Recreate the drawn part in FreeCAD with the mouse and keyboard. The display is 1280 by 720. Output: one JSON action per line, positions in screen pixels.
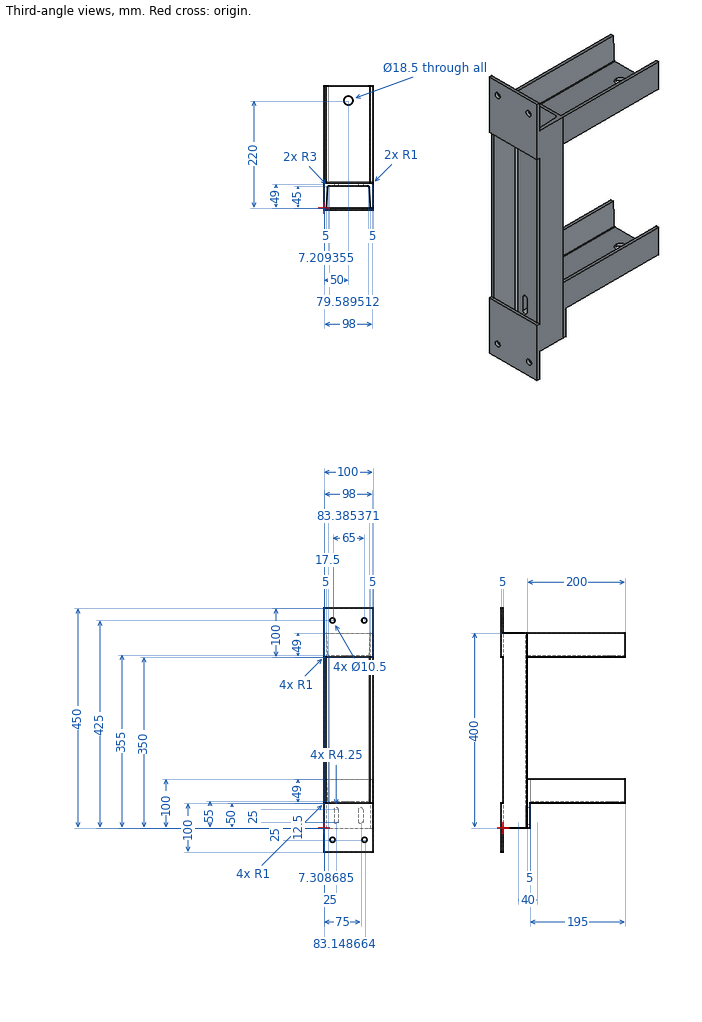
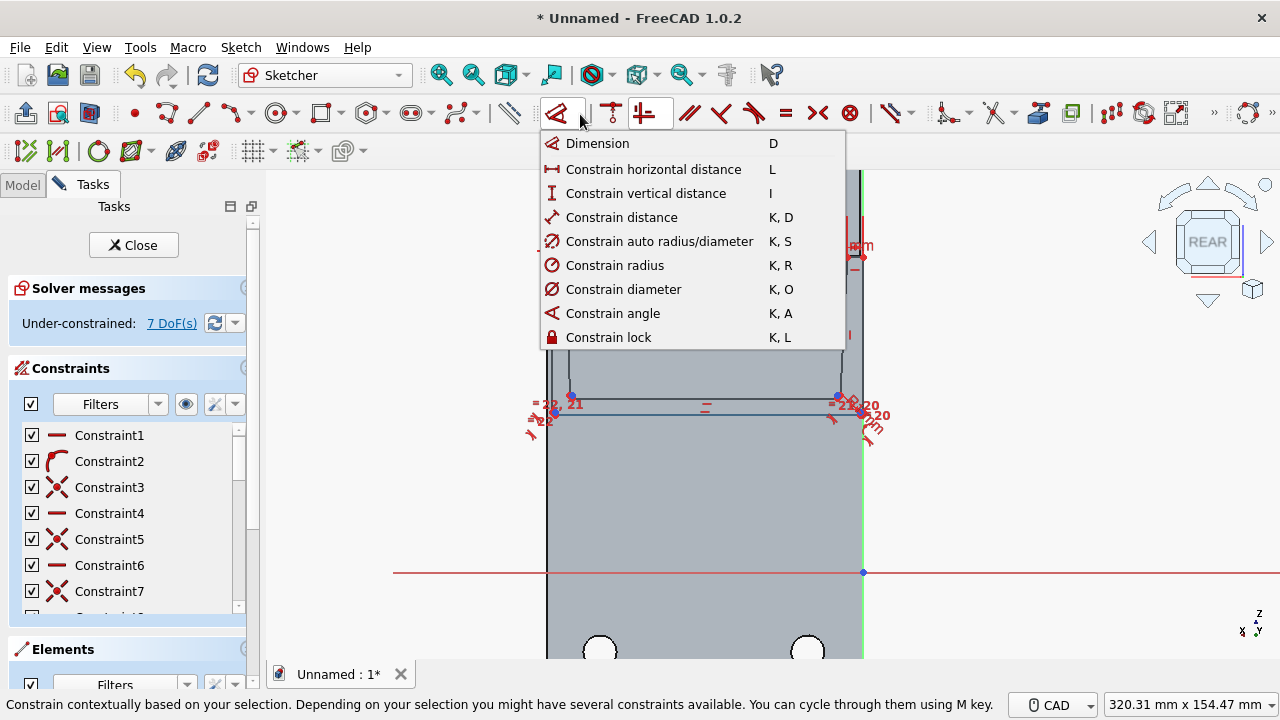
{"action": "left_click", "coordinate": [693, 169]}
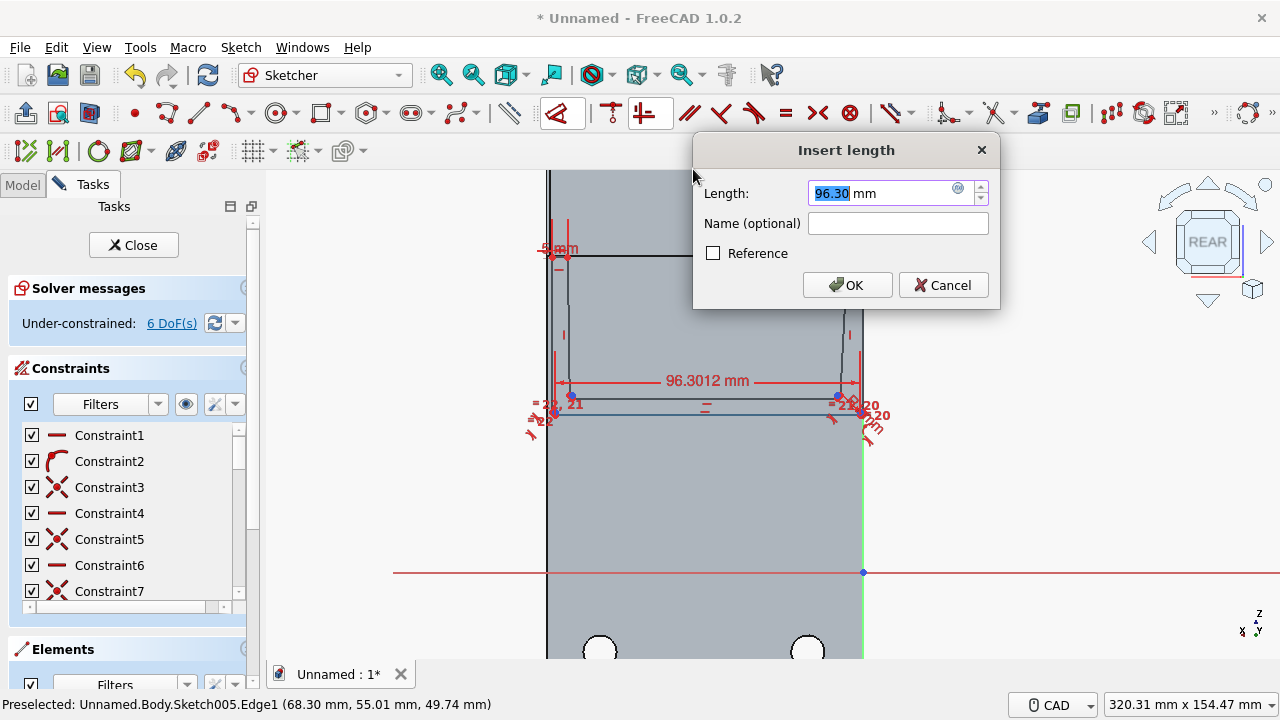
{"action": "type", "text": "98"}
{"action": "key", "text": "Return"}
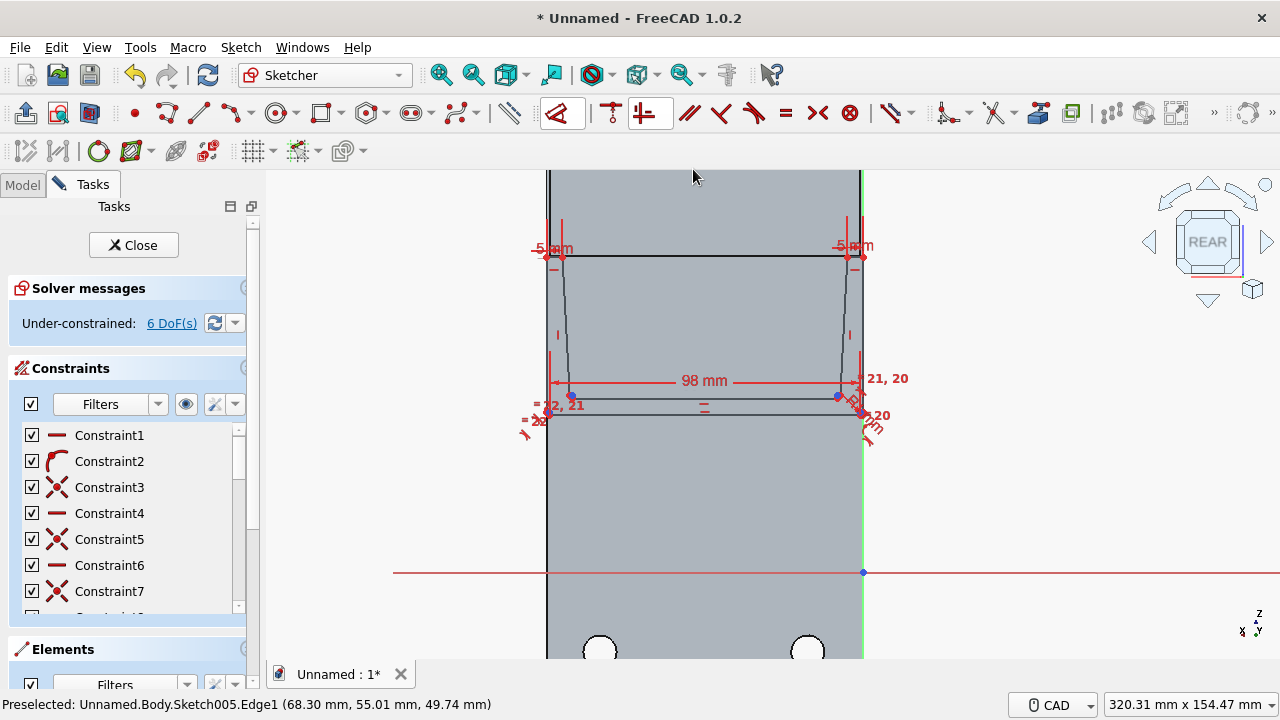
{"action": "left_click", "coordinate": [863, 366]}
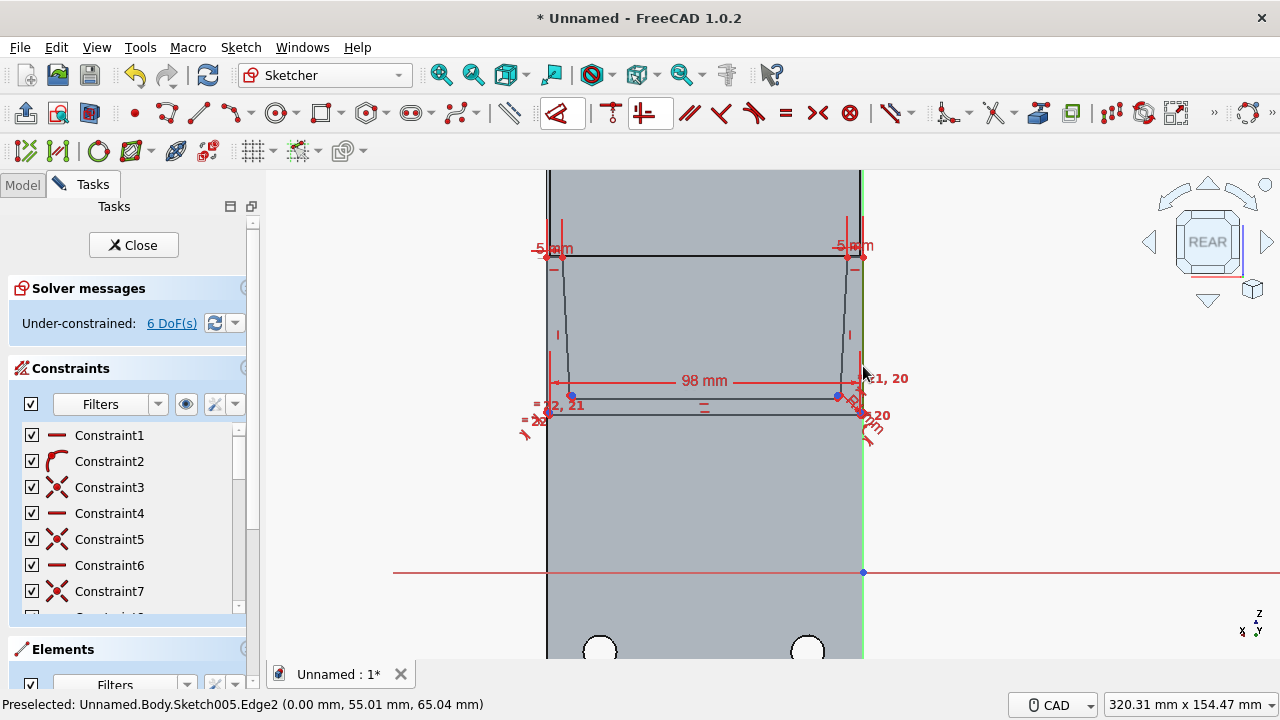
{"action": "key", "text": "i"}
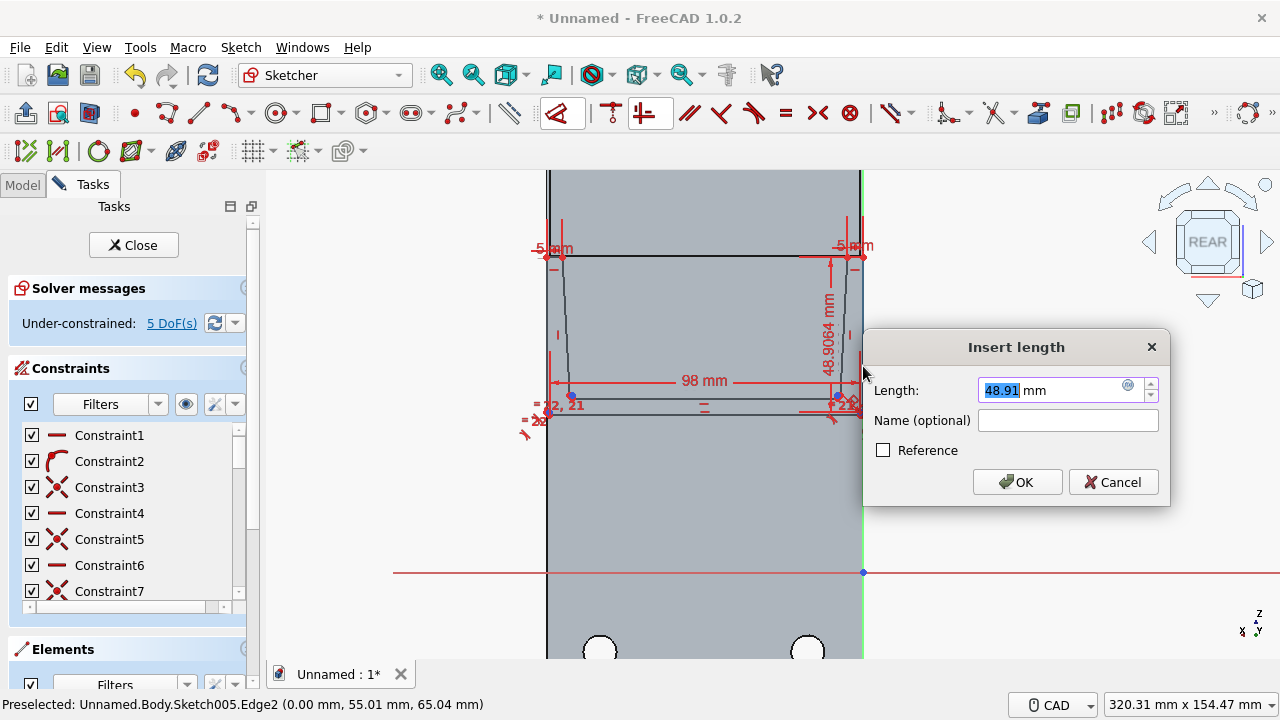
{"action": "type", "text": "49"}
{"action": "key", "text": "Return"}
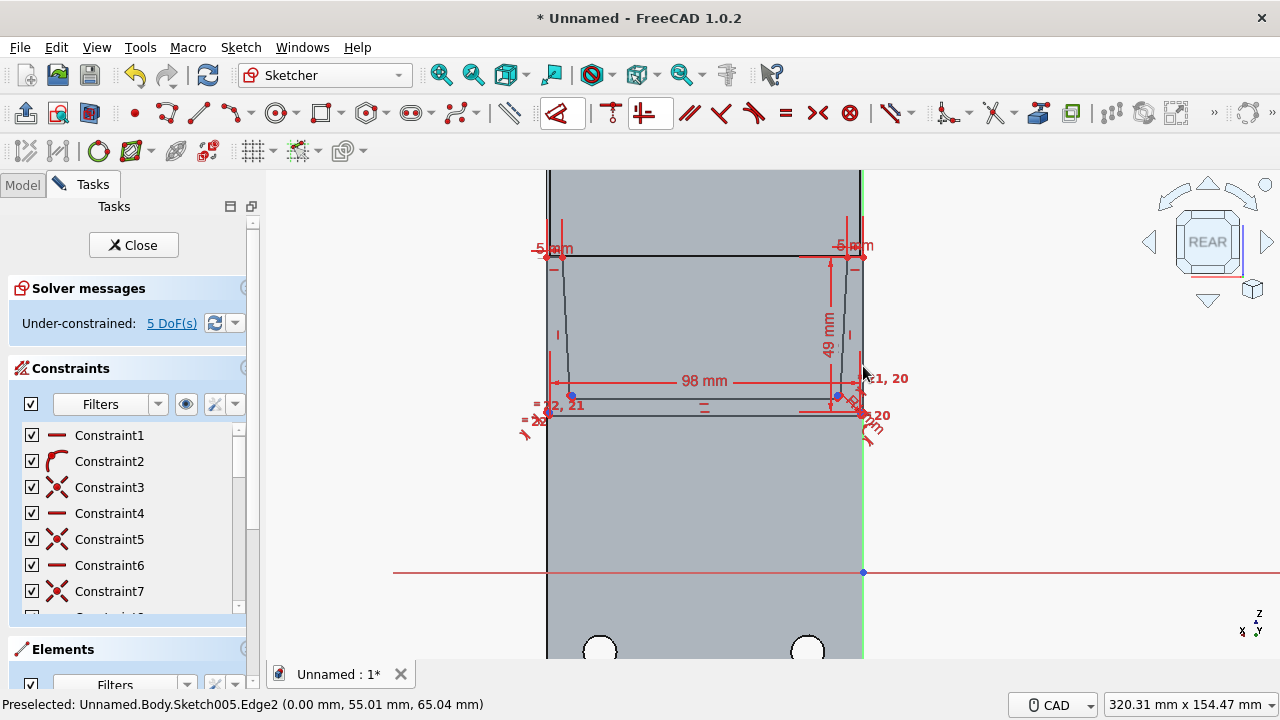
{"action": "left_click", "coordinate": [547, 304]}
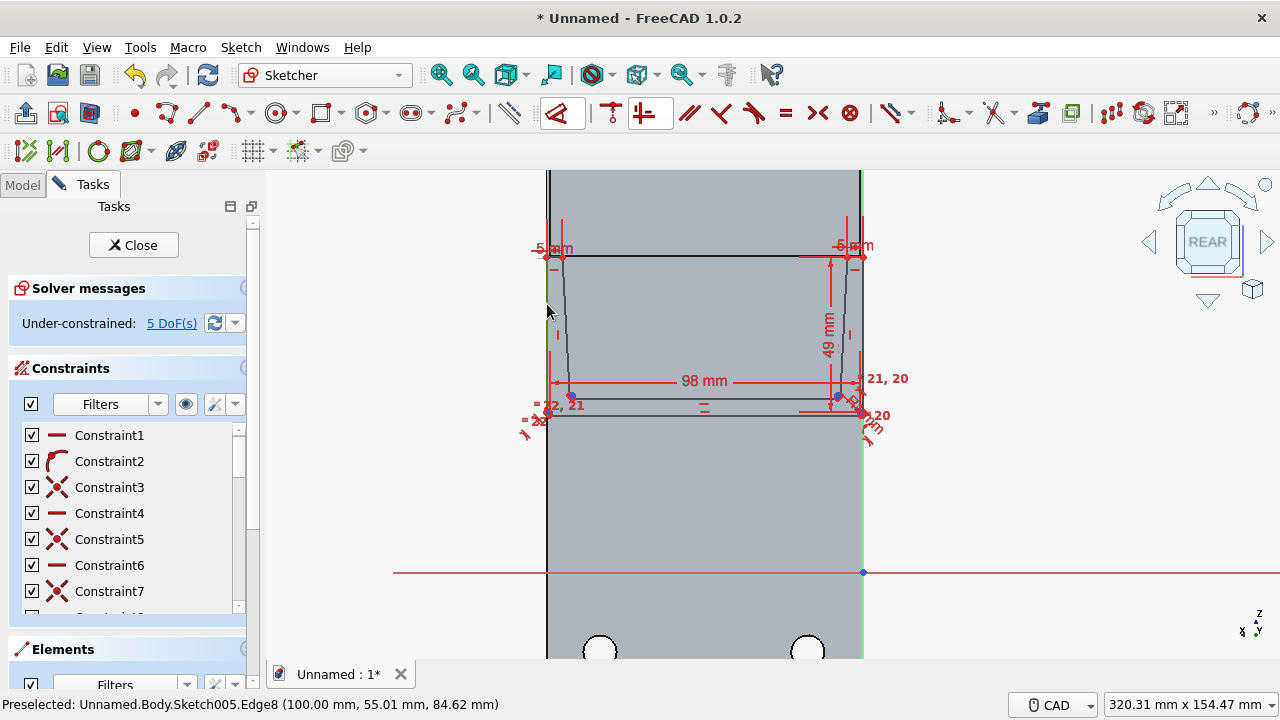
{"action": "left_click", "coordinate": [580, 114]}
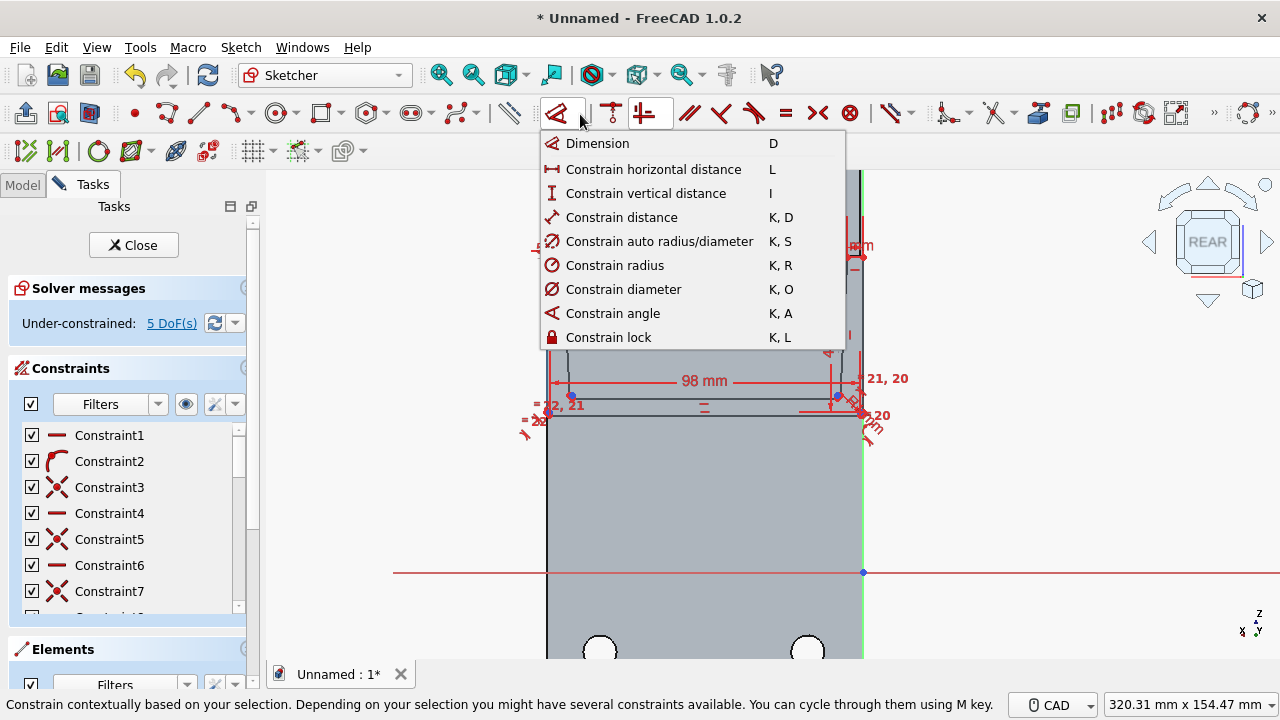
{"action": "left_click", "coordinate": [693, 193]}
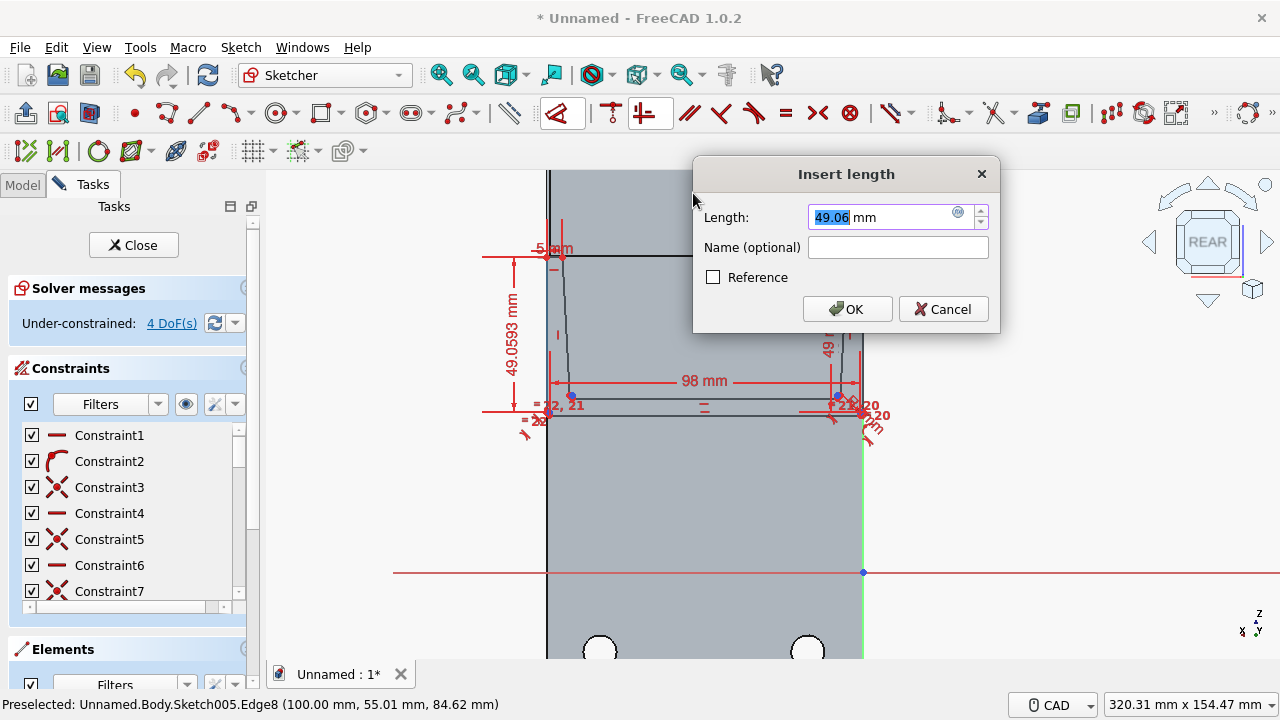
{"action": "type", "text": "49"}
{"action": "key", "text": "Return"}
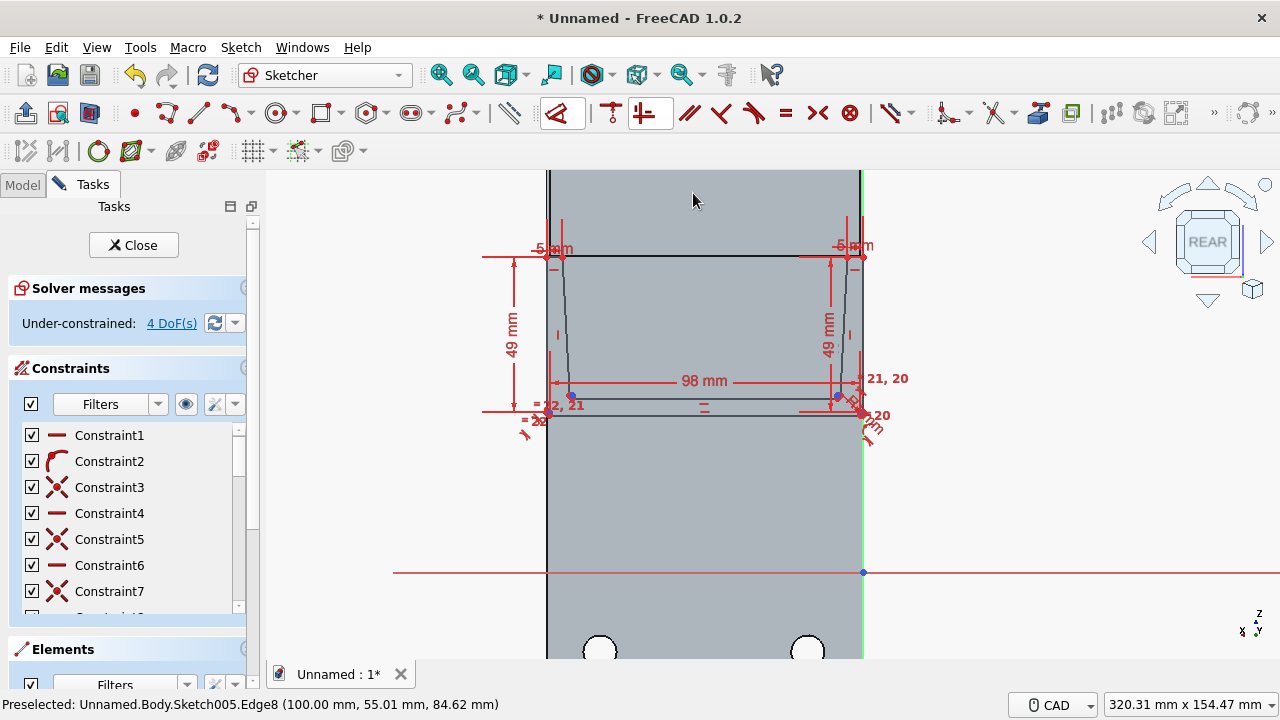
{"action": "scroll", "coordinate": [550, 416], "scroll_direction": "up", "scroll_amount": 7}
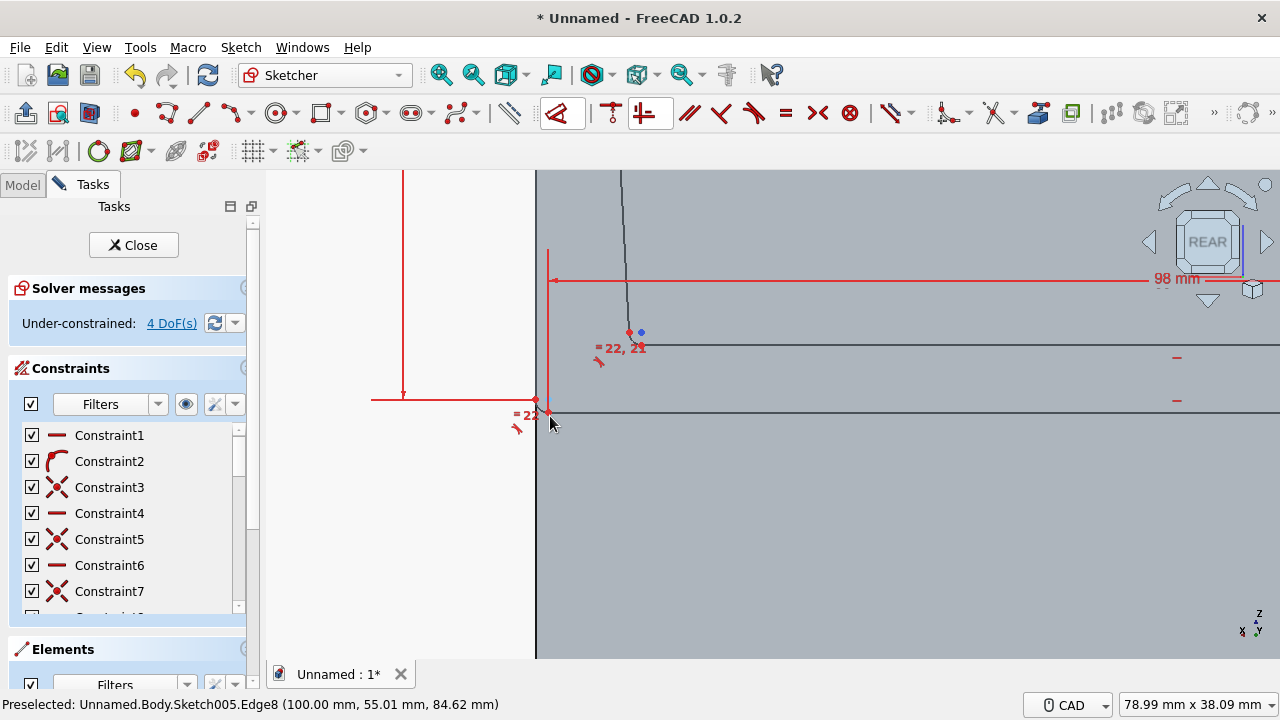
{"action": "left_click", "coordinate": [548, 413]}